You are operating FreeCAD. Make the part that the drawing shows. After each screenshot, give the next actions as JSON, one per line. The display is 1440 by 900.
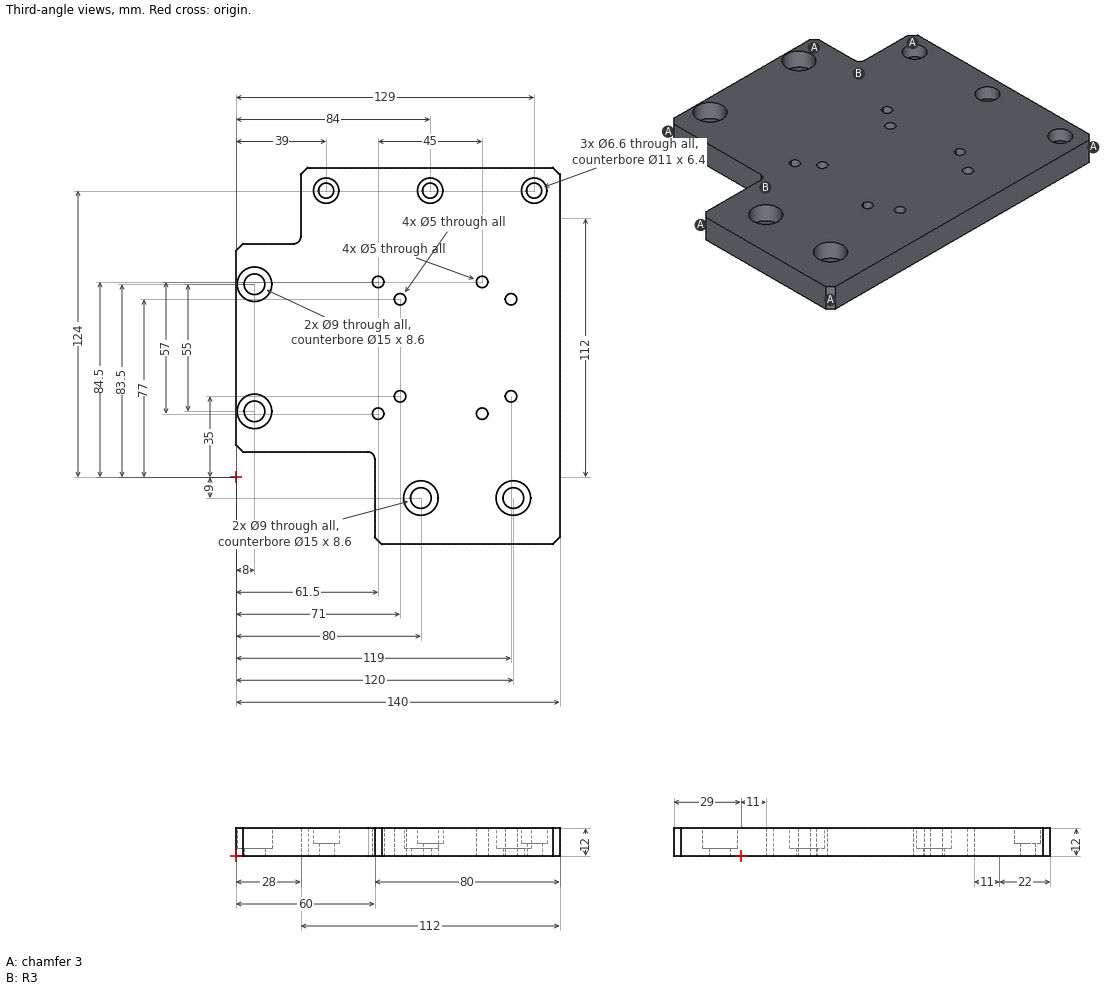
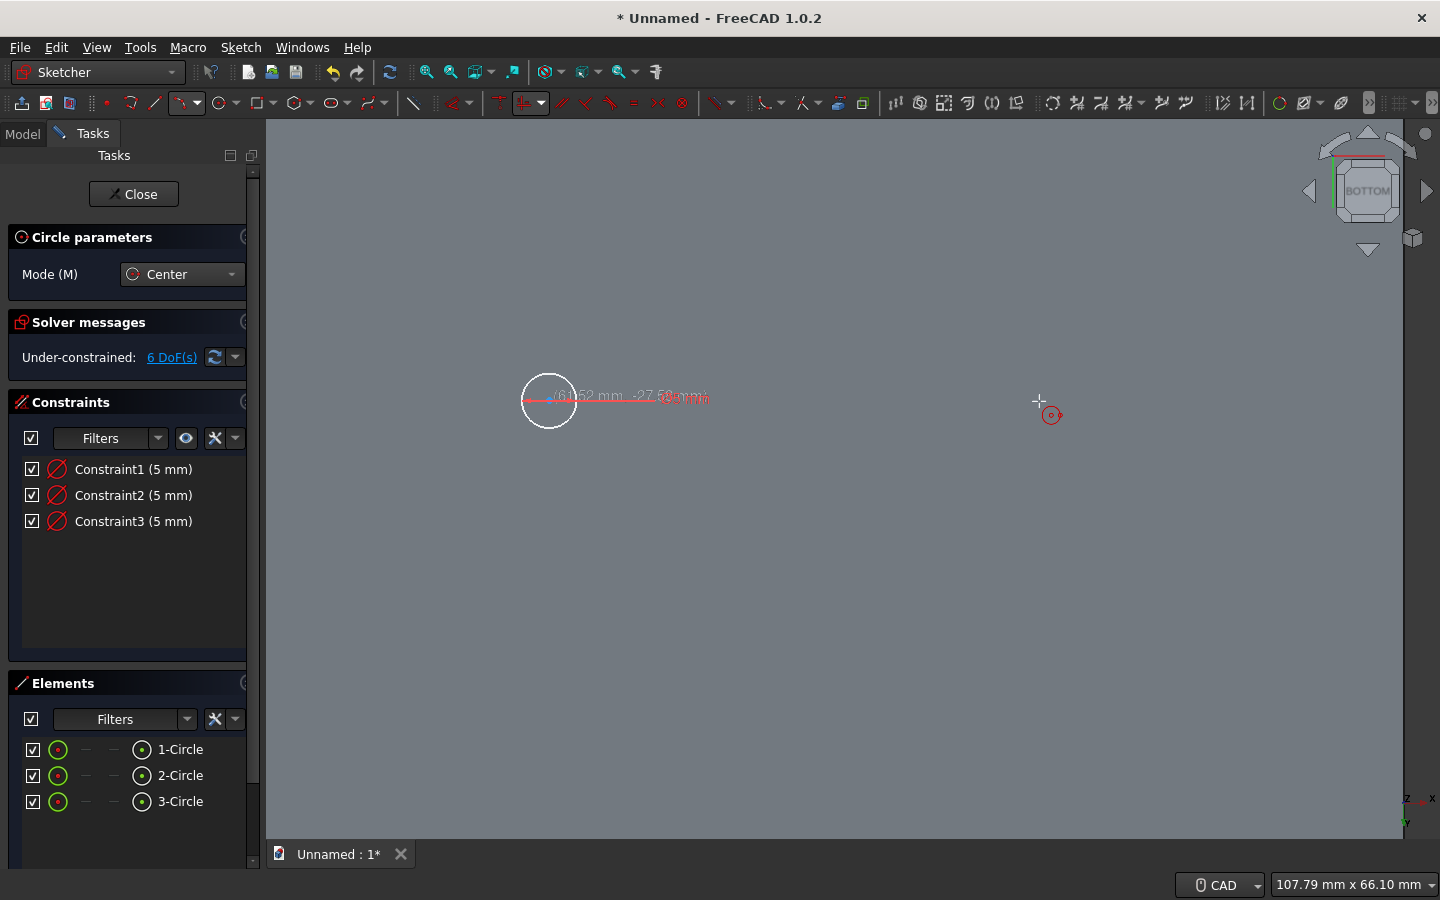
{"action": "left_click", "coordinate": [1039, 400]}
{"action": "mouse_move", "coordinate": [1058, 381]}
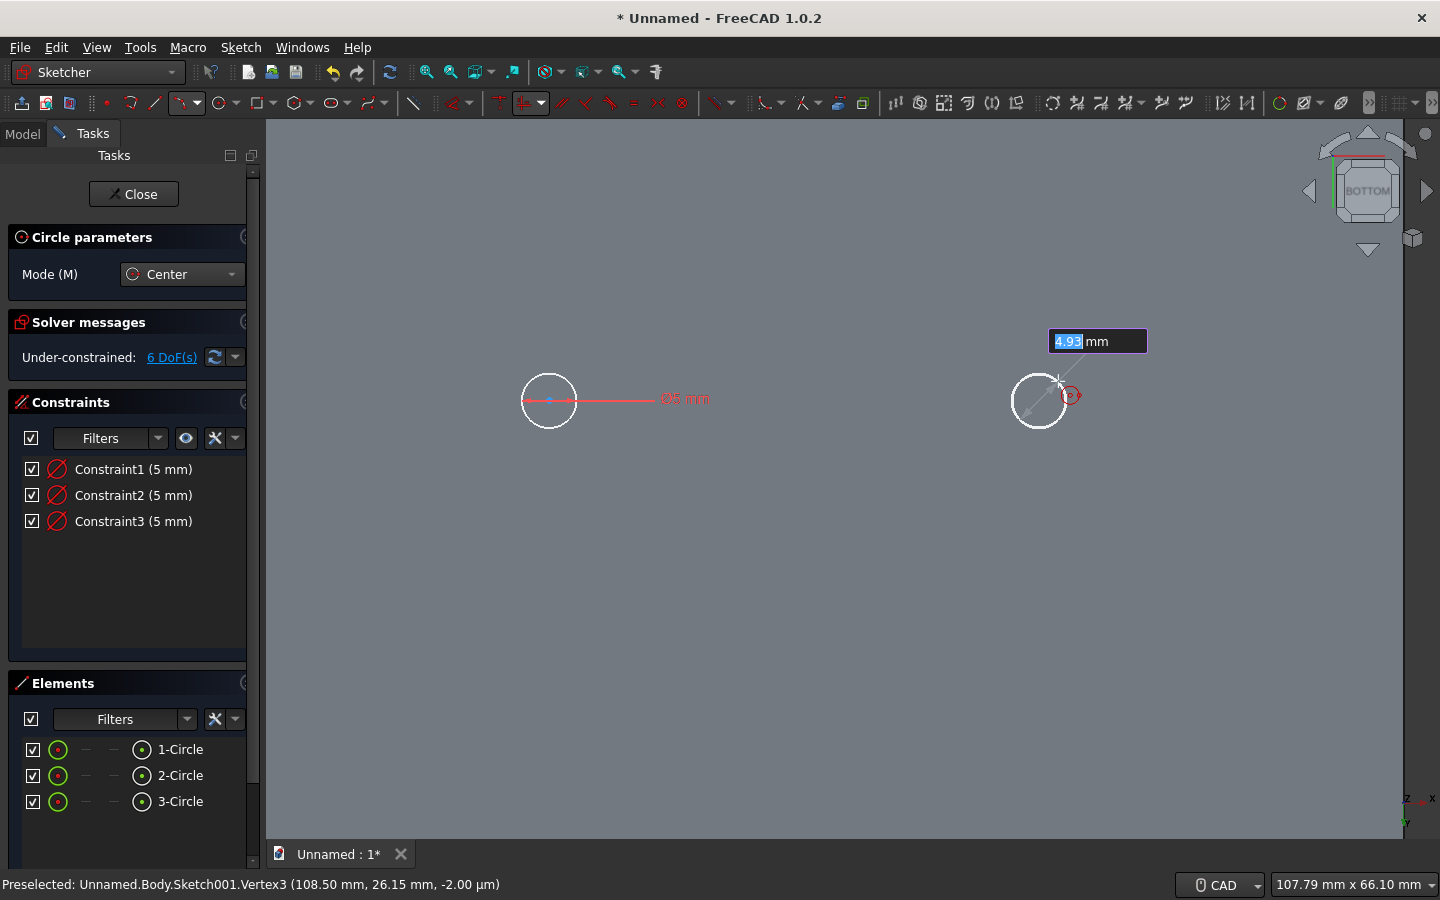
{"action": "type", "text": "5"}
{"action": "key", "text": "Return"}
{"action": "key", "text": "Escape"}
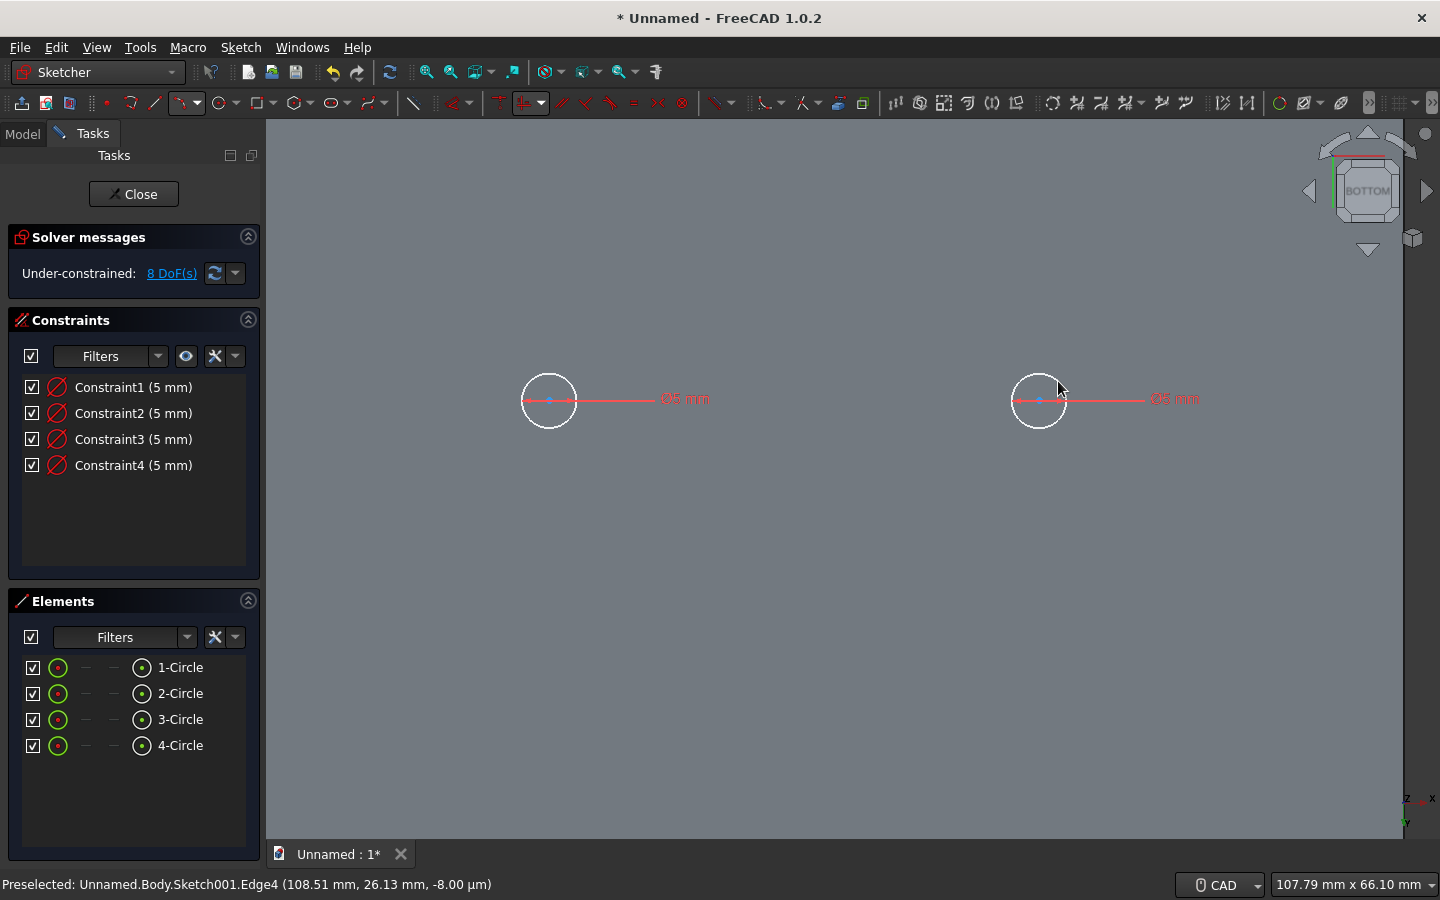
{"action": "scroll", "coordinate": [1039, 401], "scroll_direction": "down", "scroll_amount": 4}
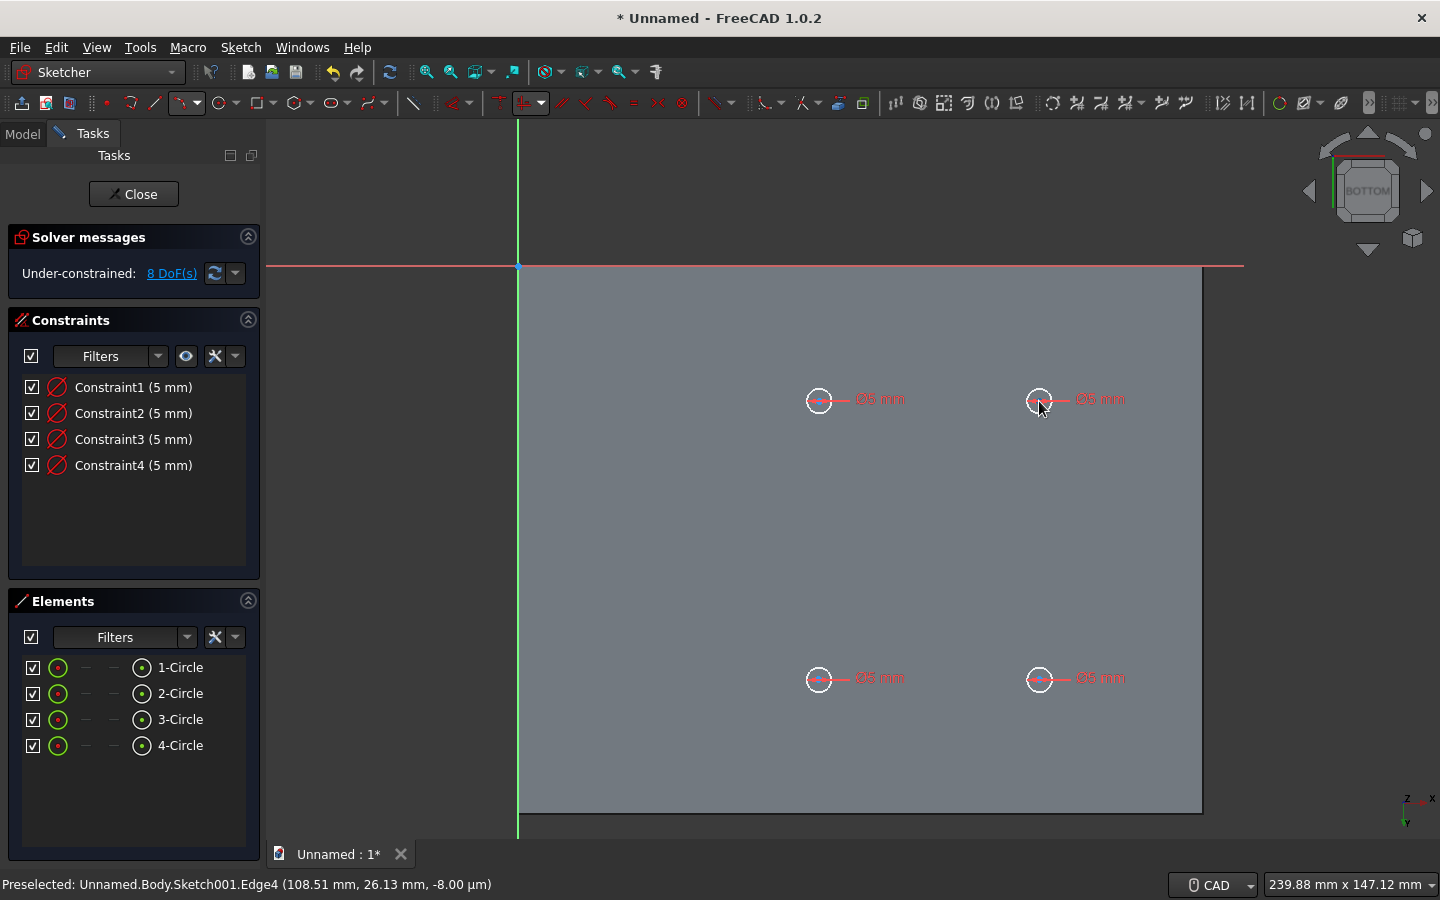
{"action": "left_click", "coordinate": [1040, 680]}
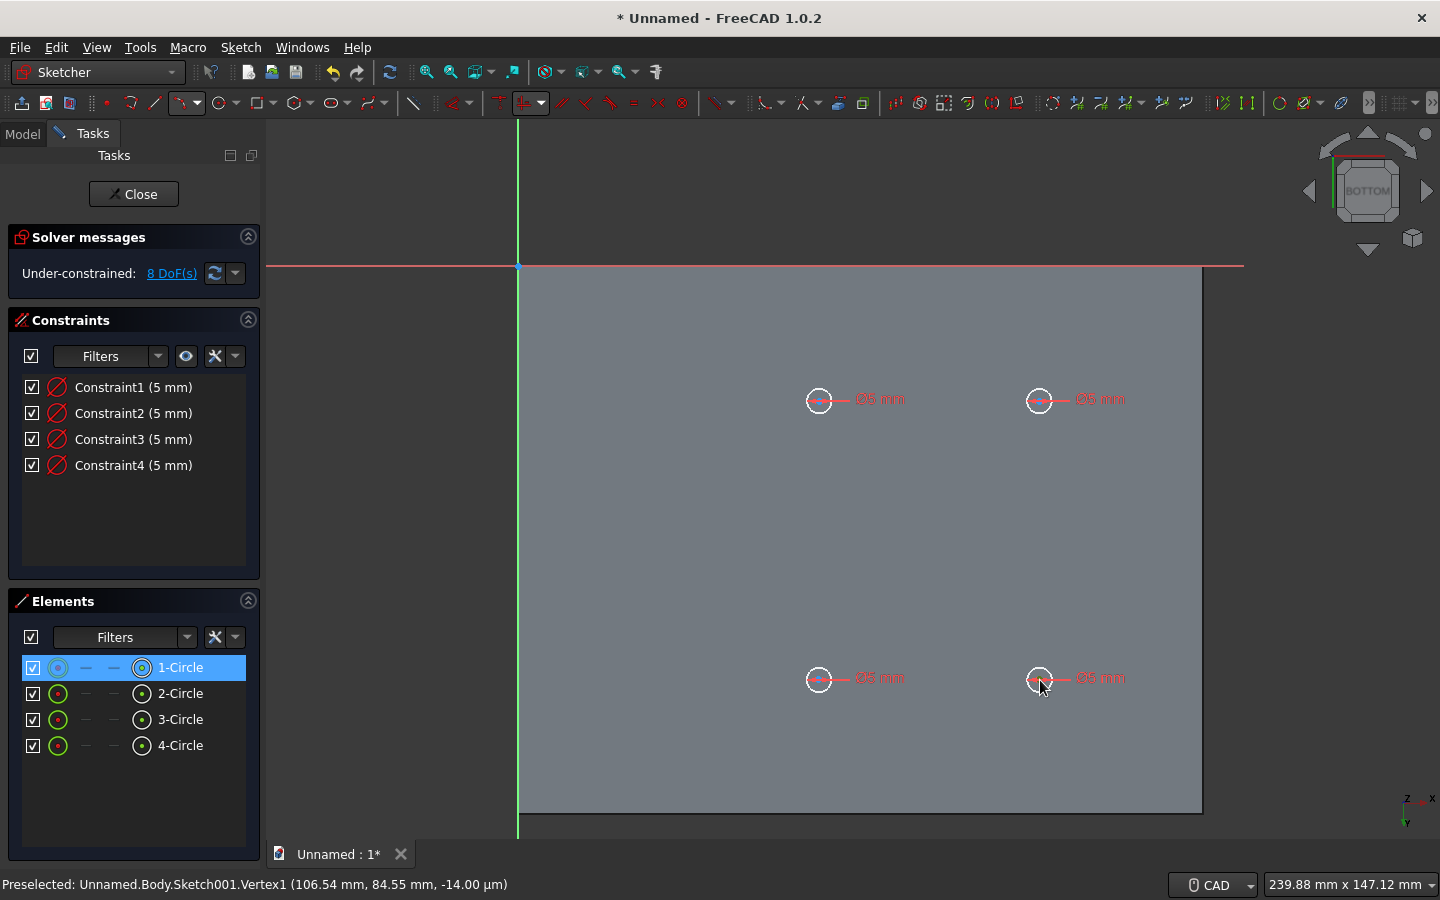
{"action": "left_click", "coordinate": [819, 680]}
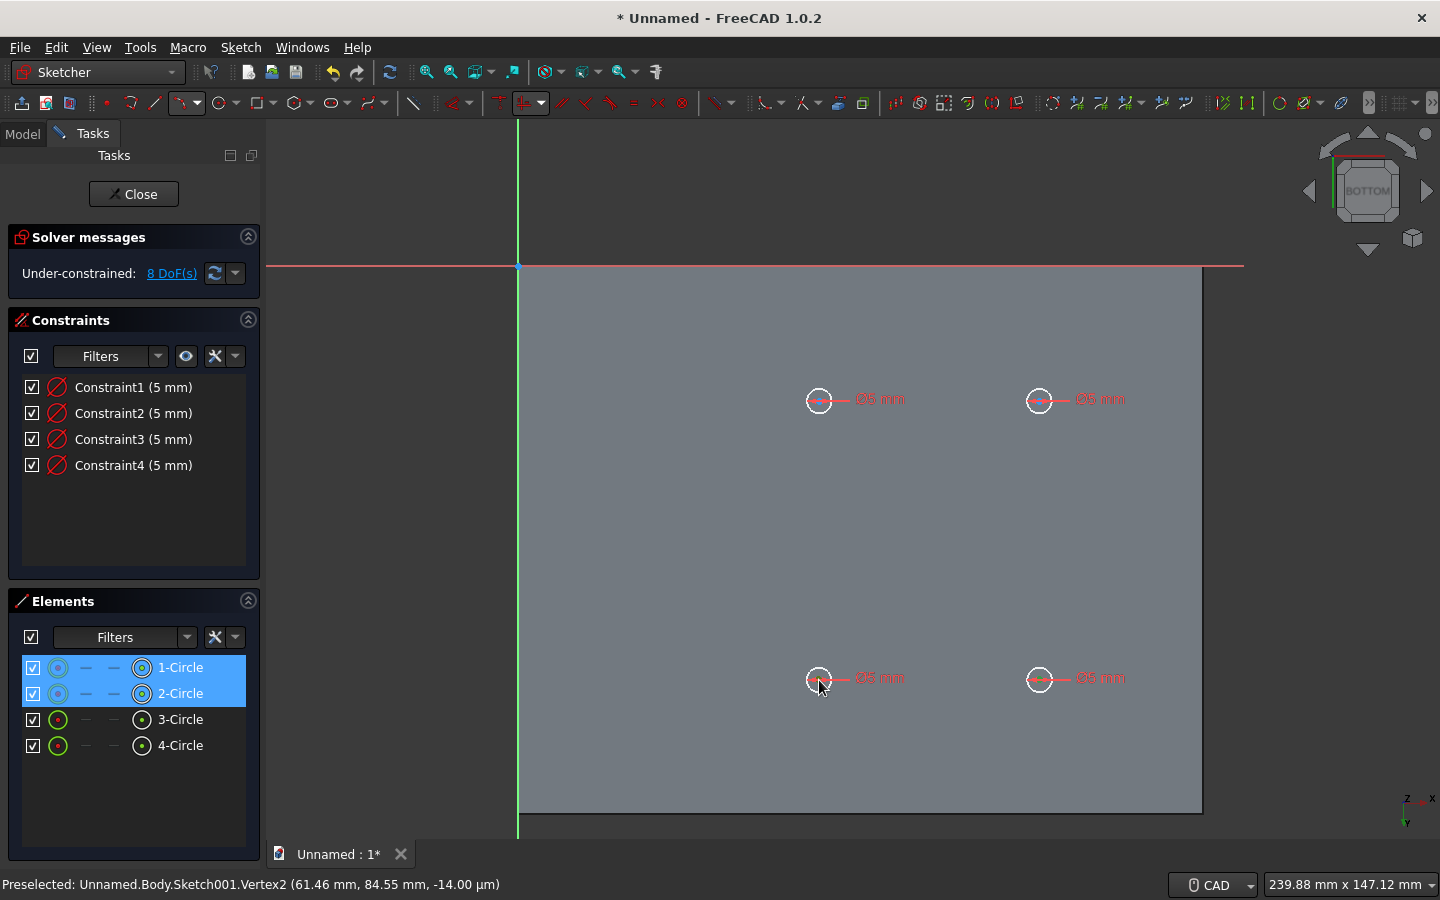
{"action": "left_click", "coordinate": [472, 104]}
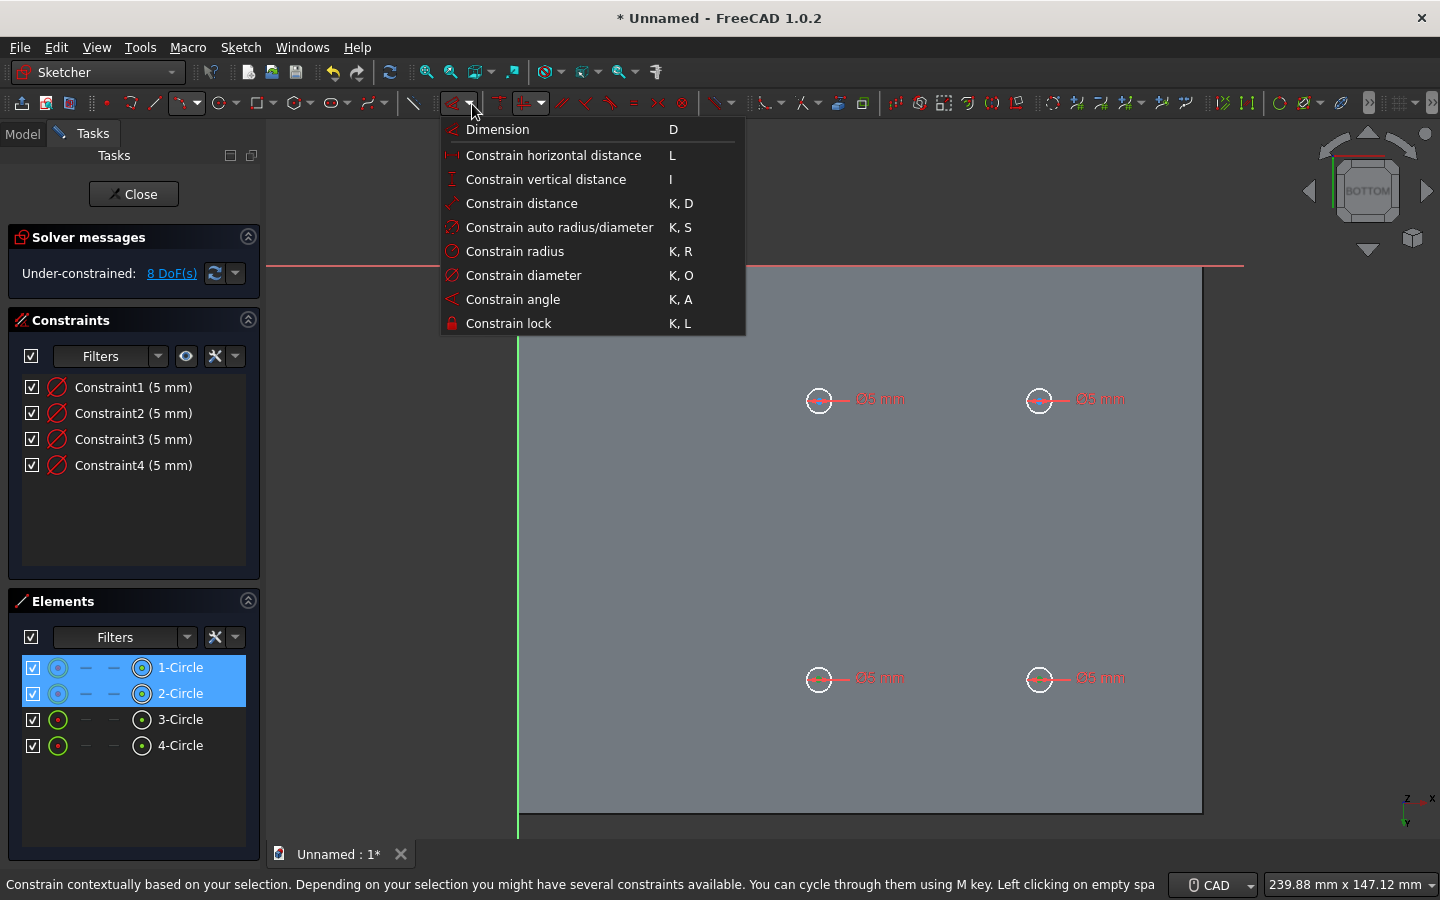
{"action": "left_click", "coordinate": [593, 155]}